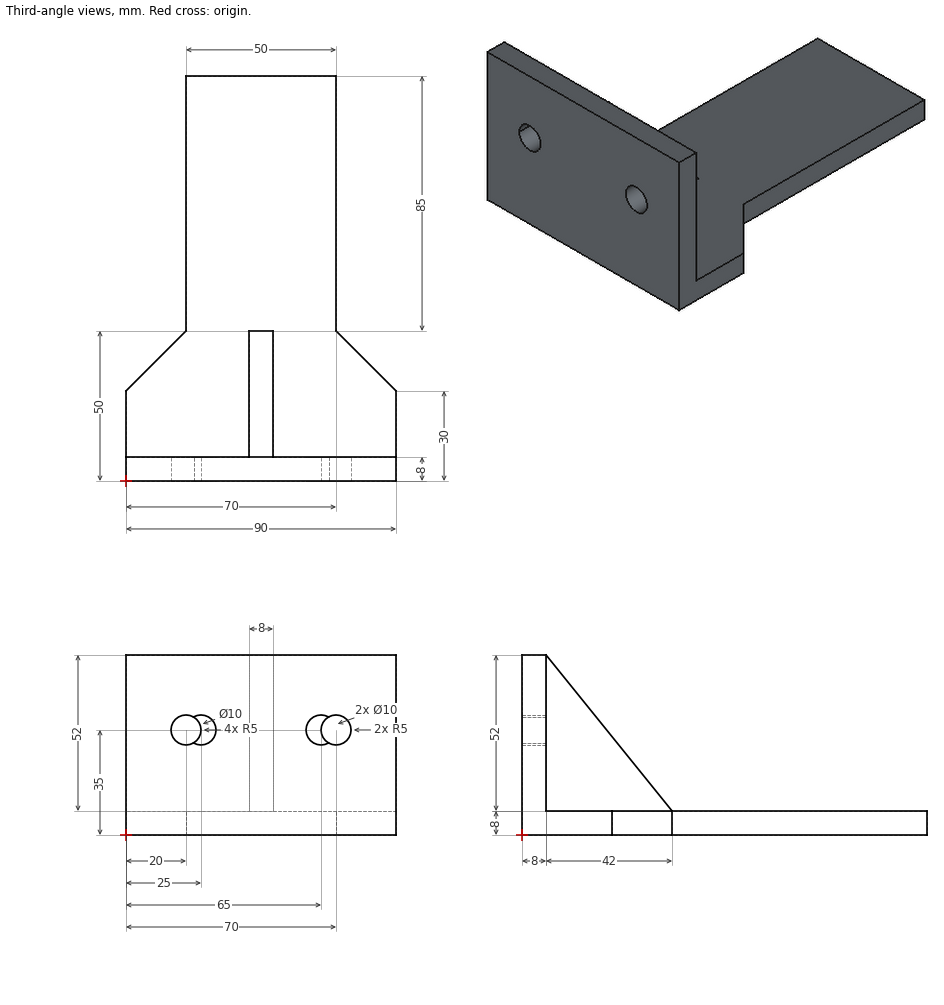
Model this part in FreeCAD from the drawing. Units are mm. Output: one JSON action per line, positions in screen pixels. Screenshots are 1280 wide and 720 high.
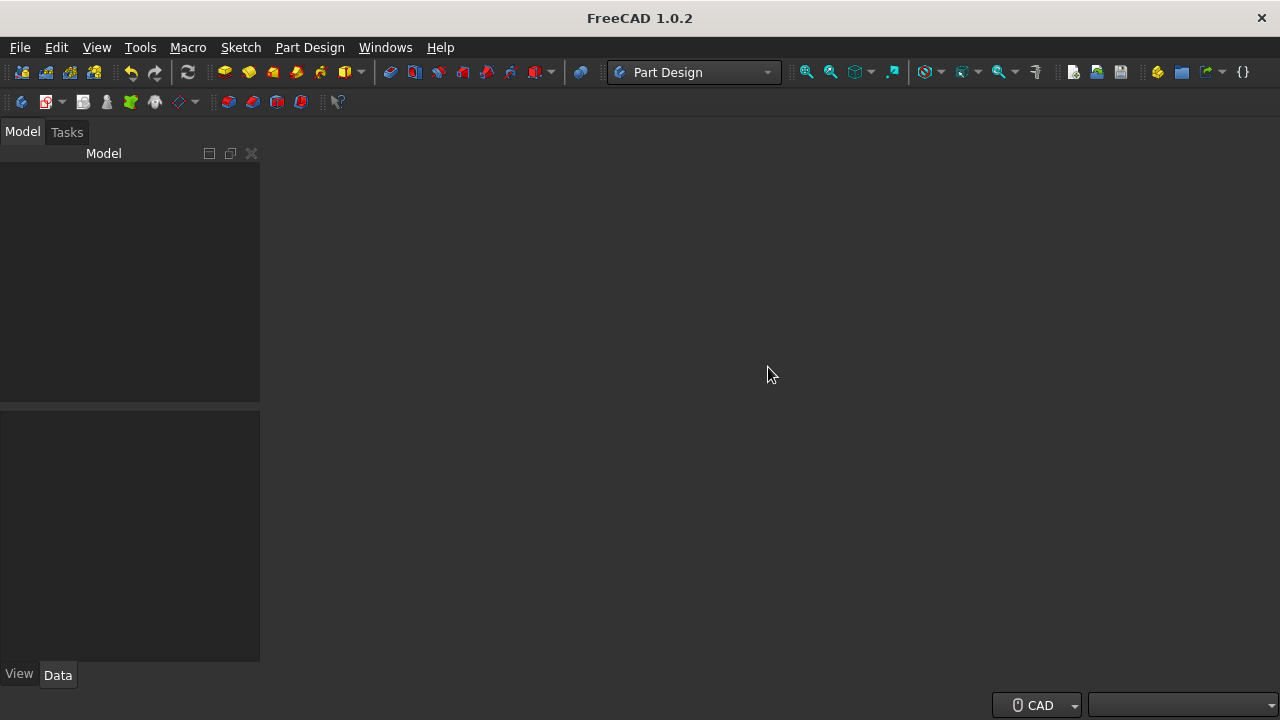
{"action": "left_click", "coordinate": [1074, 72]}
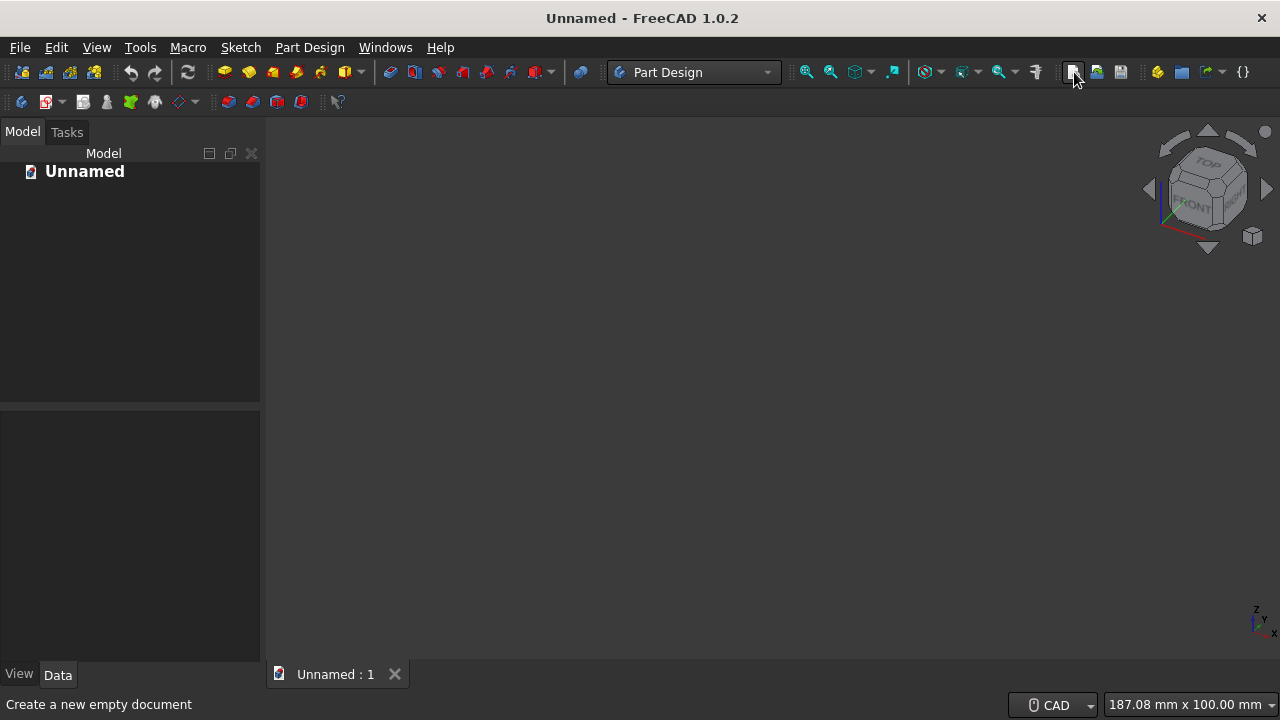
{"action": "left_click", "coordinate": [46, 102]}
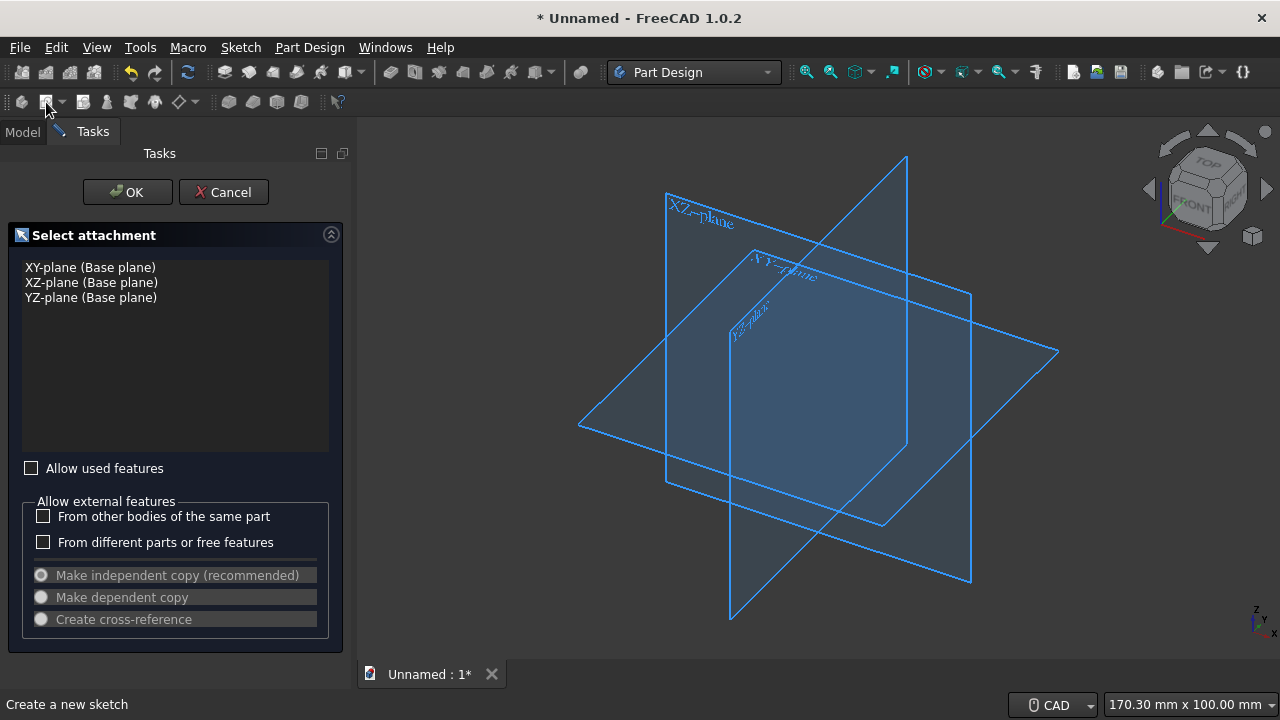
{"action": "left_click", "coordinate": [82, 268]}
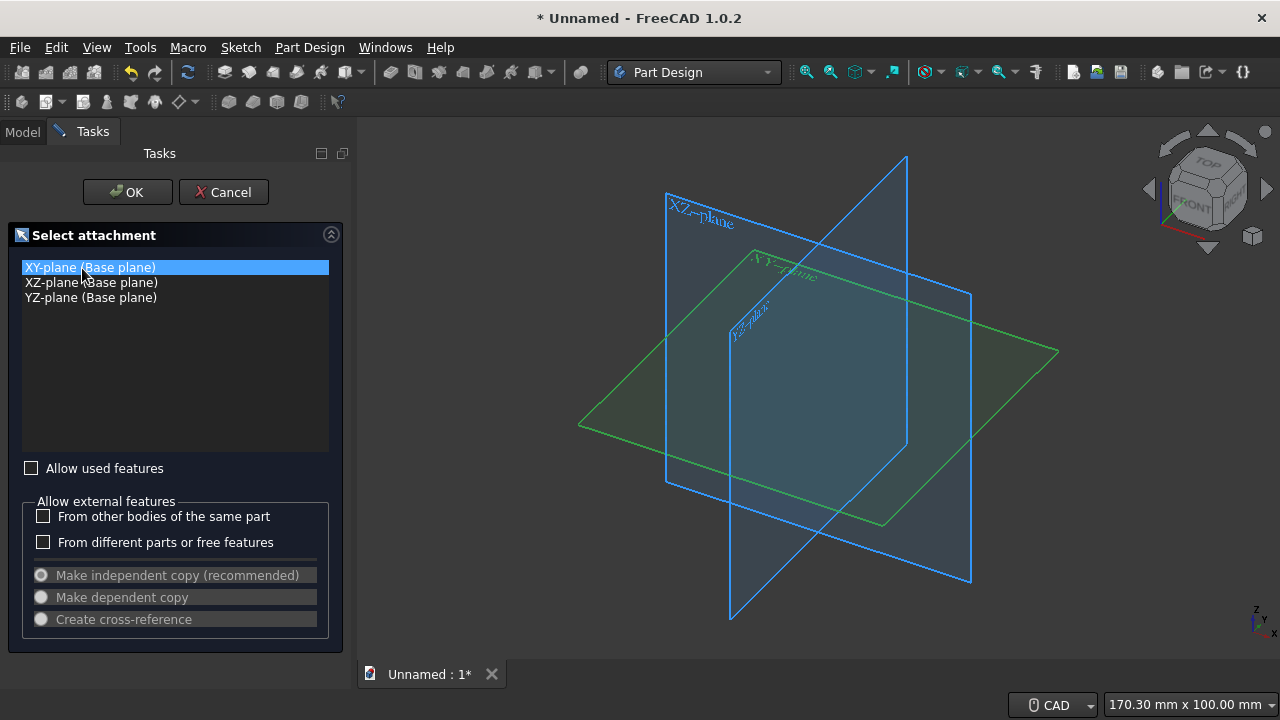
{"action": "left_click", "coordinate": [128, 192]}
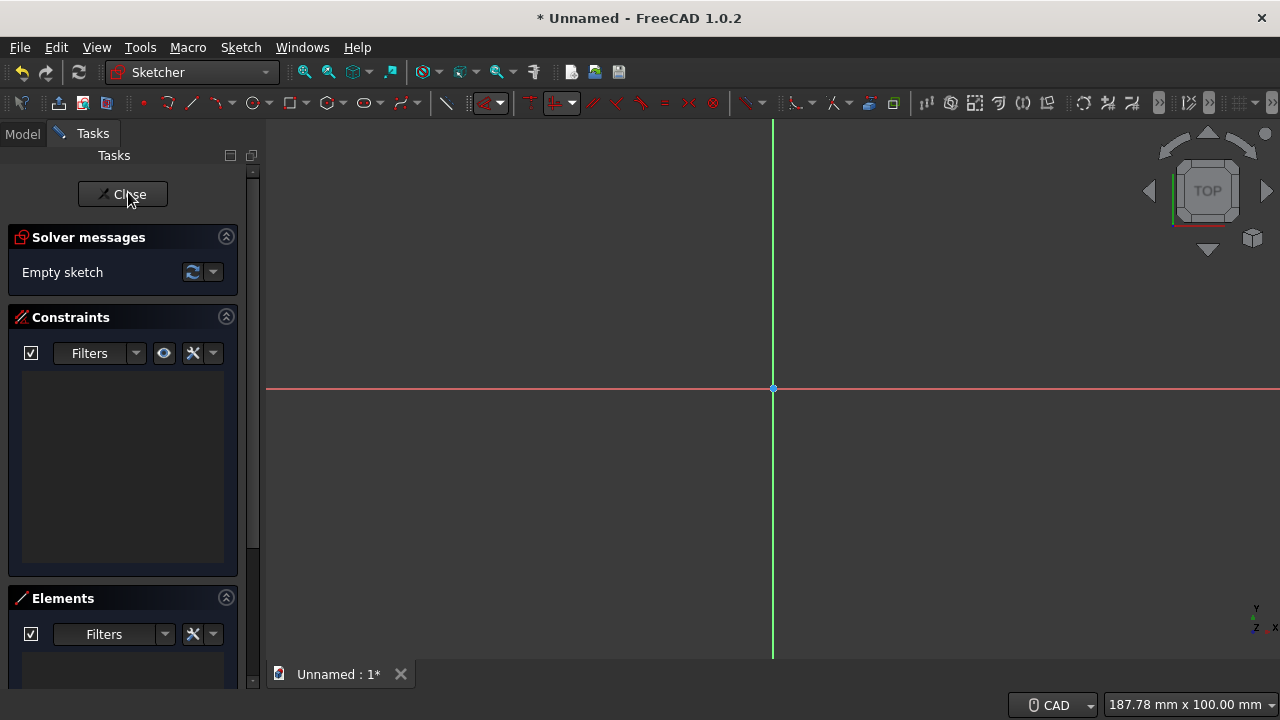
{"action": "scroll", "coordinate": [450, 631], "scroll_direction": "down", "scroll_amount": 4}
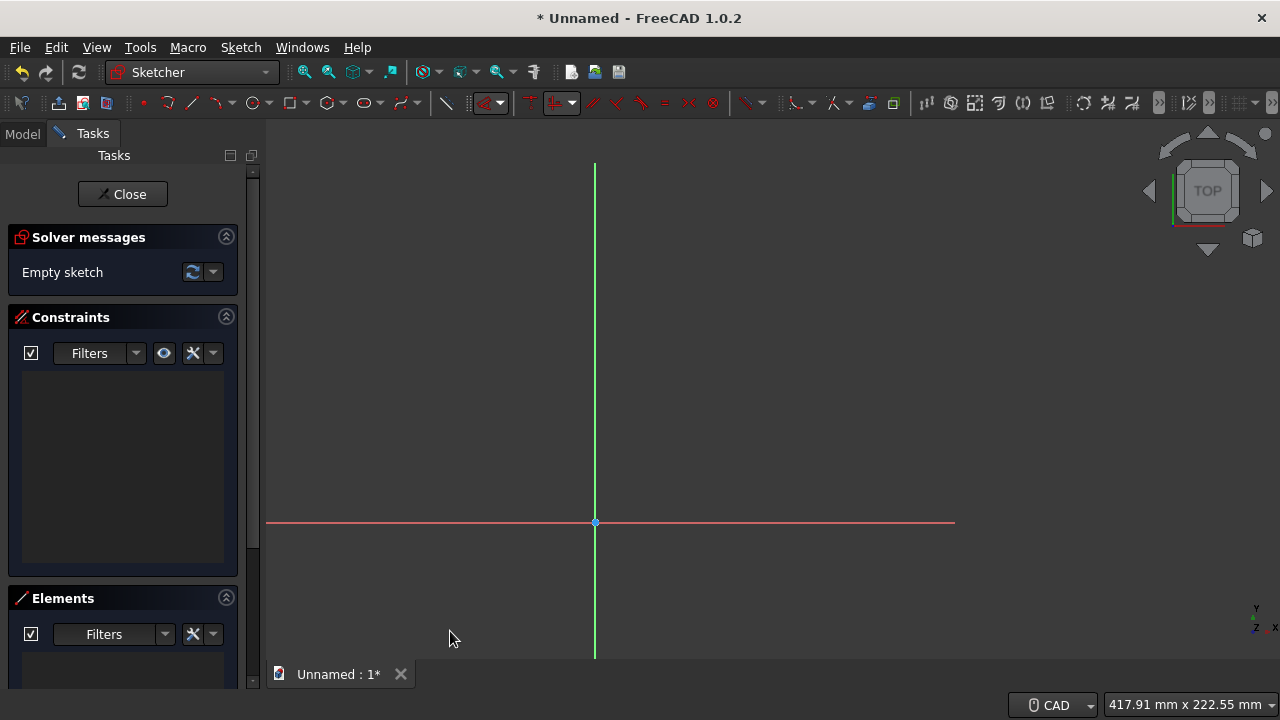
{"action": "left_click", "coordinate": [168, 104]}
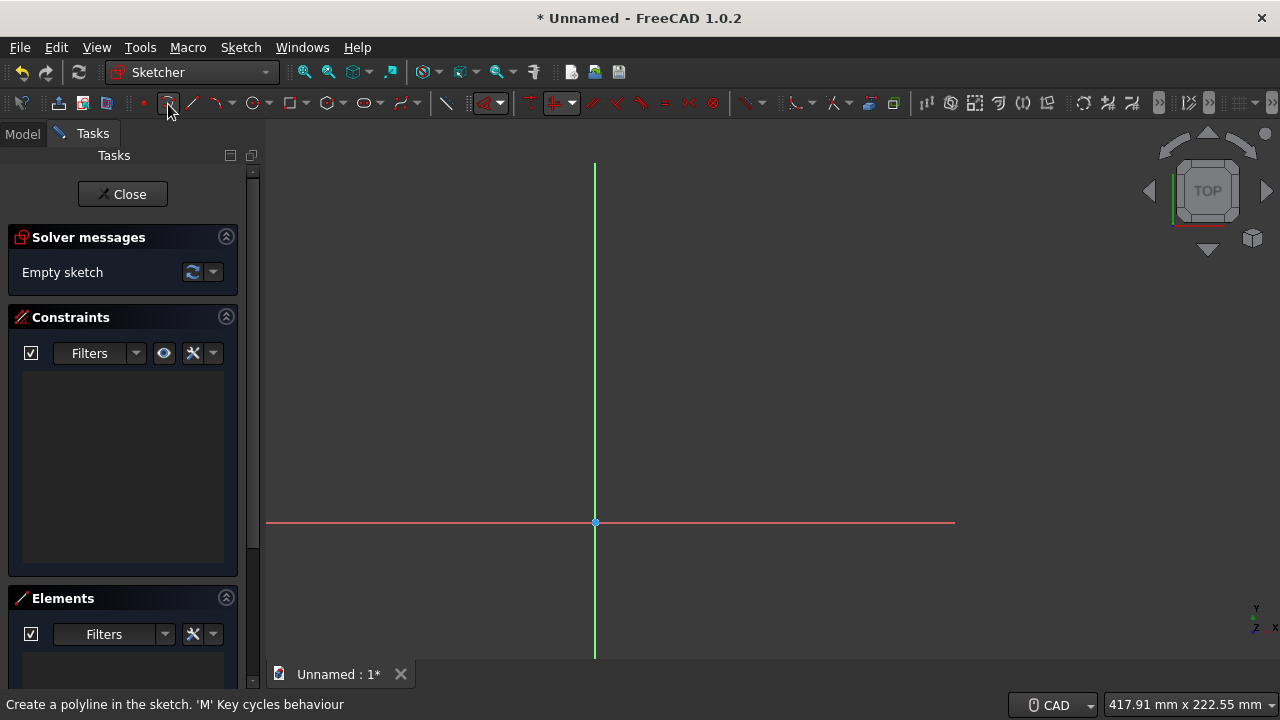
{"action": "left_click", "coordinate": [595, 523]}
{"action": "left_click", "coordinate": [814, 514]}
{"action": "left_click", "coordinate": [814, 450]}
{"action": "left_click", "coordinate": [765, 401]}
{"action": "left_click", "coordinate": [765, 195]}
{"action": "left_click", "coordinate": [644, 195]}
{"action": "left_click", "coordinate": [644, 401]}
{"action": "left_click", "coordinate": [604, 450]}
{"action": "left_click", "coordinate": [595, 523]}
{"action": "key", "text": "Escape"}
{"action": "key", "text": "Escape"}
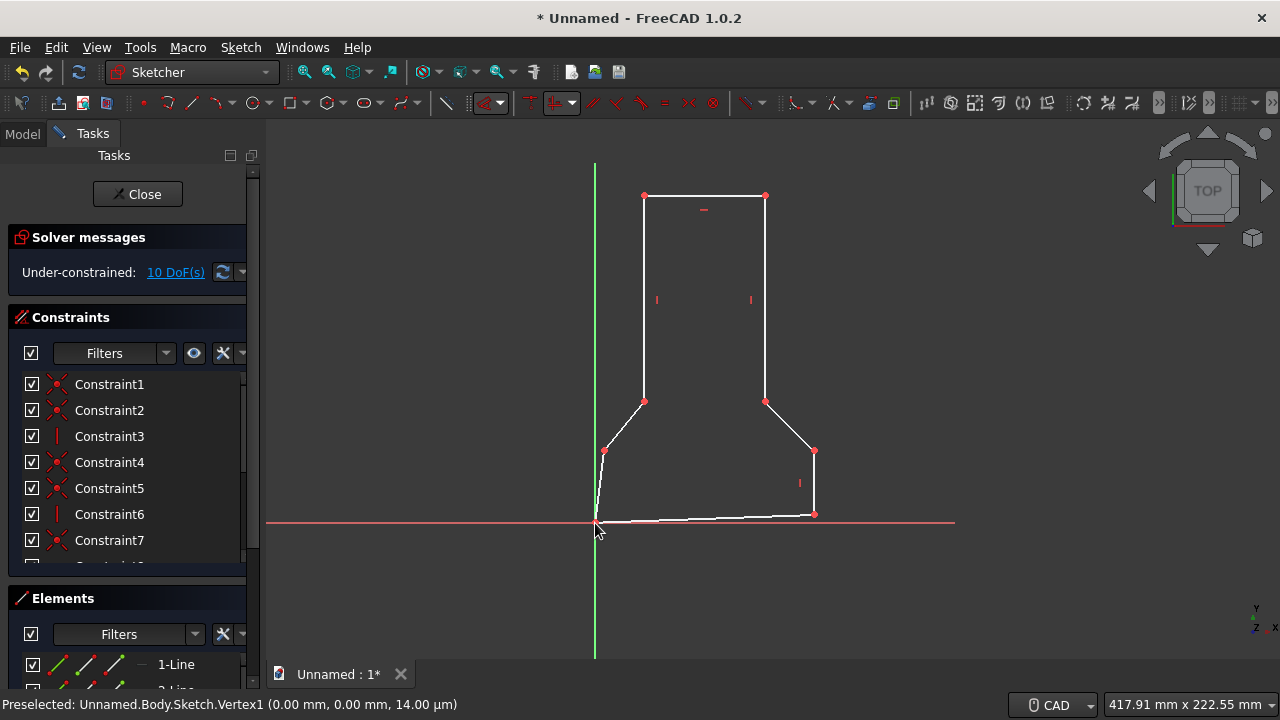
{"action": "left_click", "coordinate": [661, 520]}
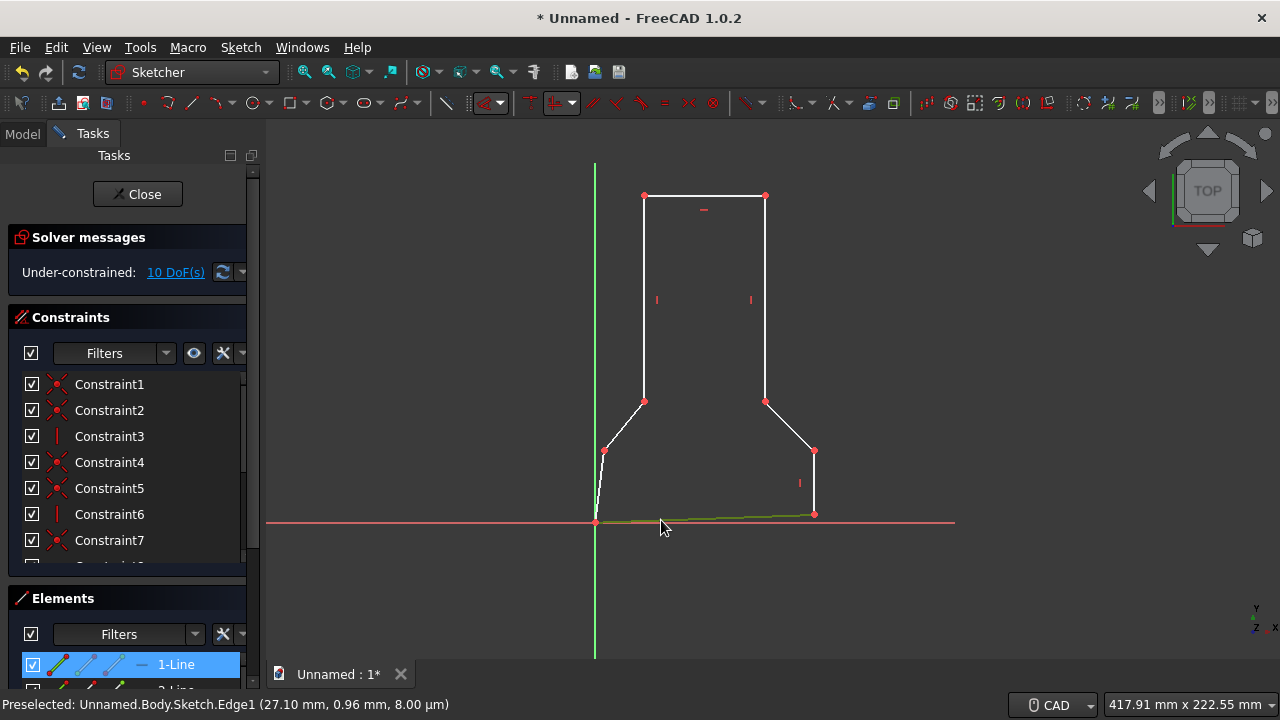
{"action": "left_click", "coordinate": [574, 104]}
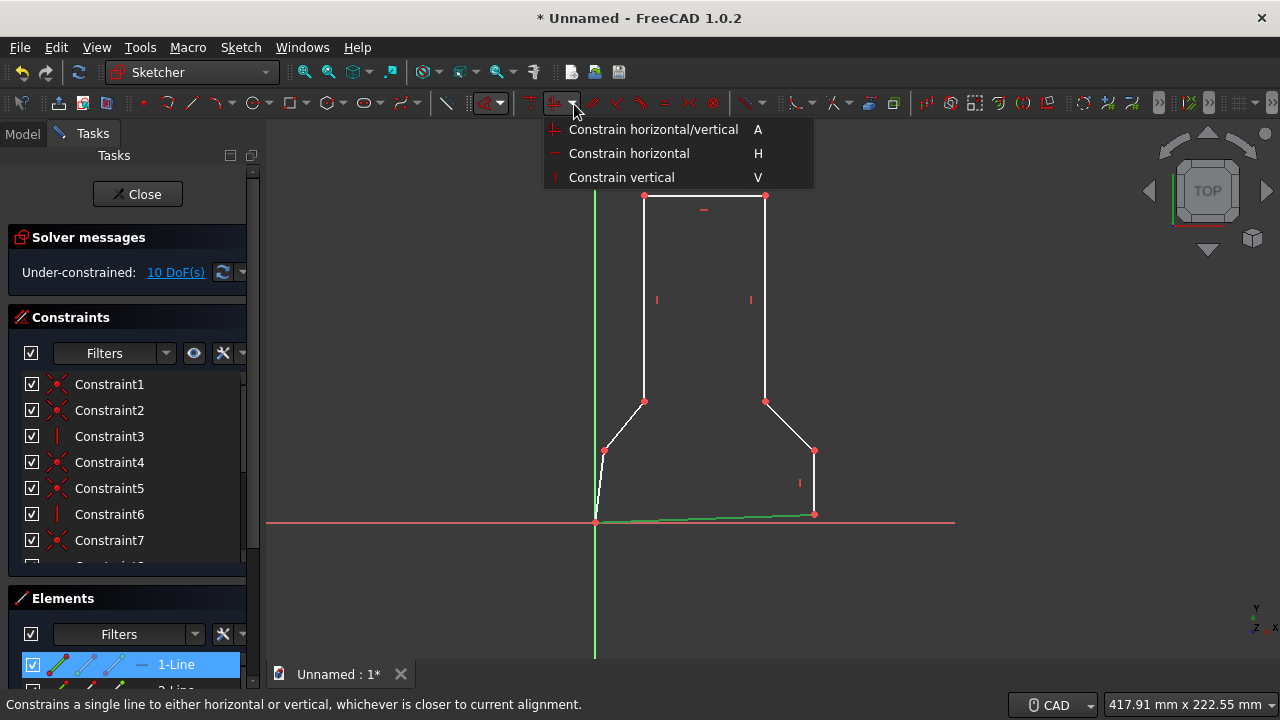
{"action": "left_click", "coordinate": [679, 153]}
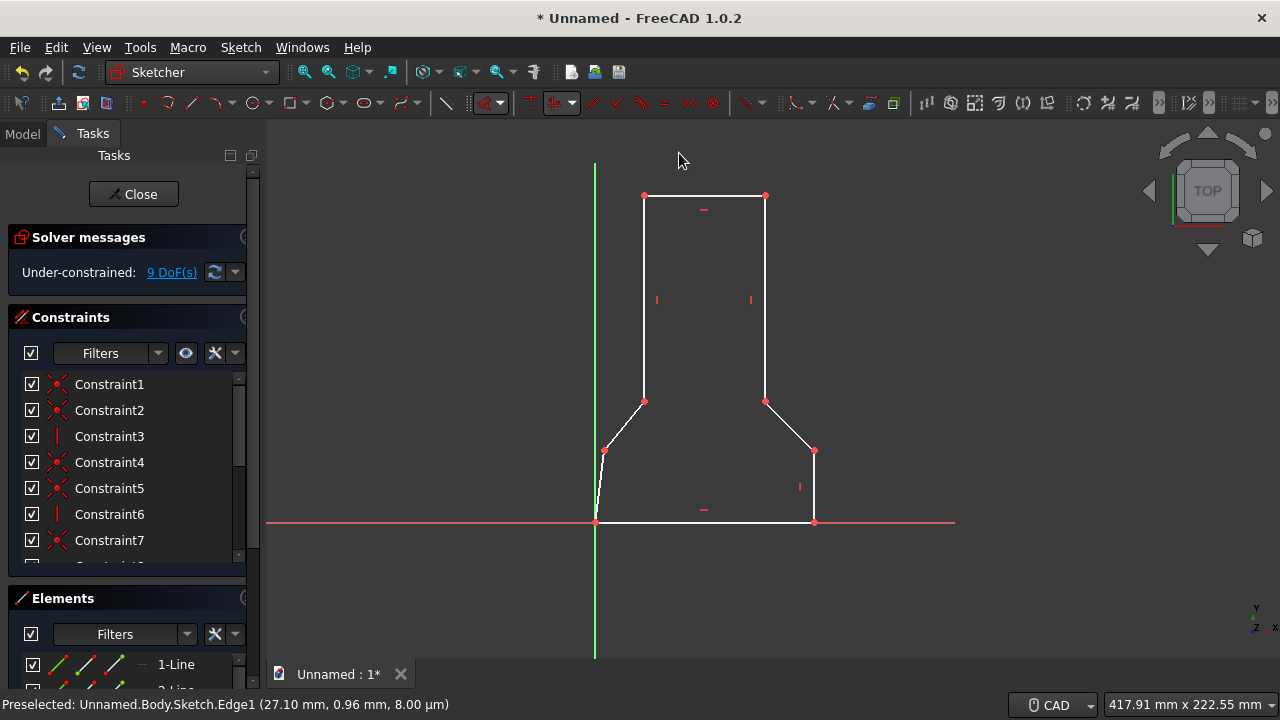
{"action": "left_click", "coordinate": [598, 501]}